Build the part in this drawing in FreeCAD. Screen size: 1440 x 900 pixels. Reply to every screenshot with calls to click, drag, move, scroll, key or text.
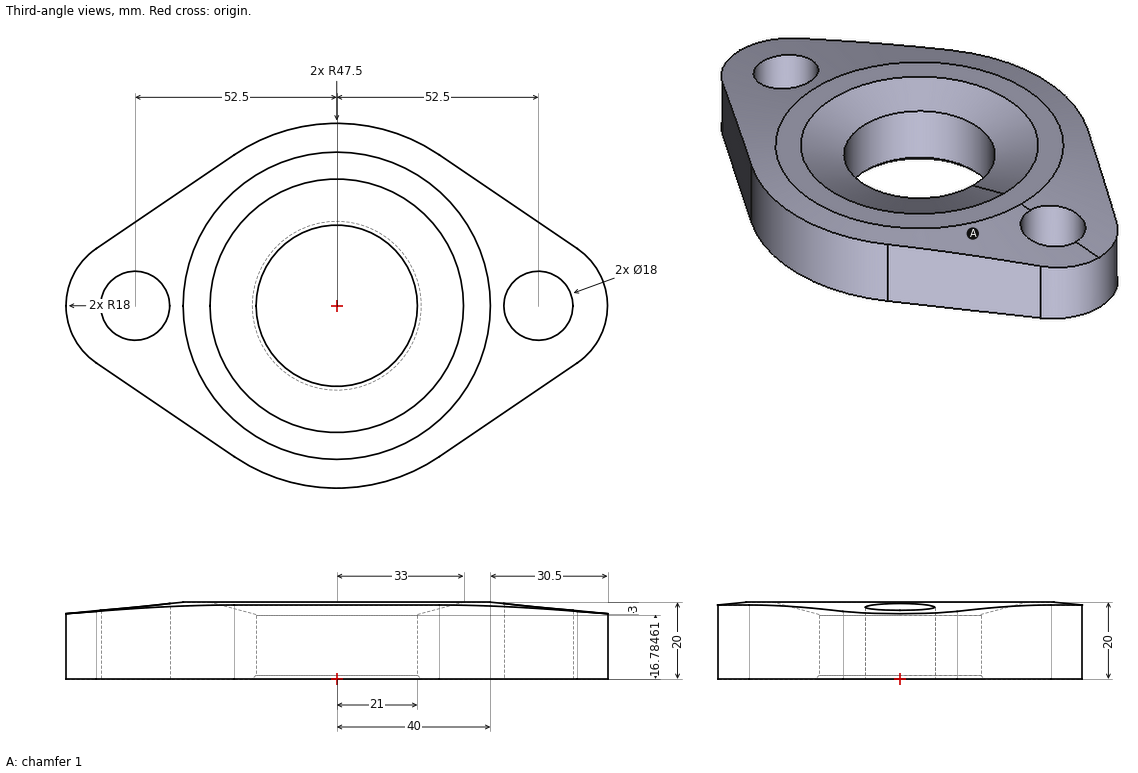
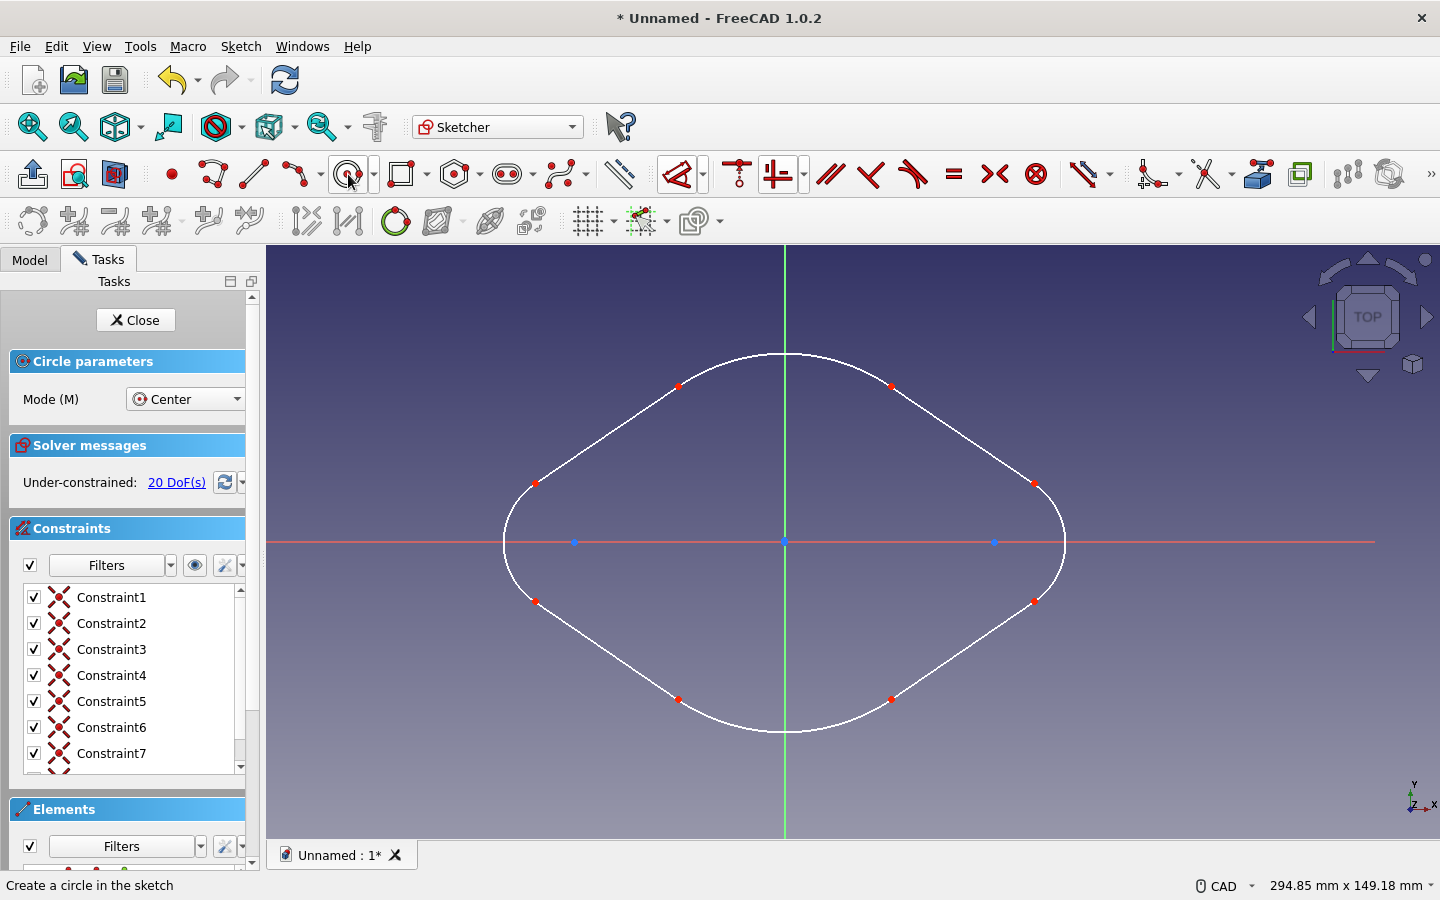
click(994, 542)
move(1019, 517)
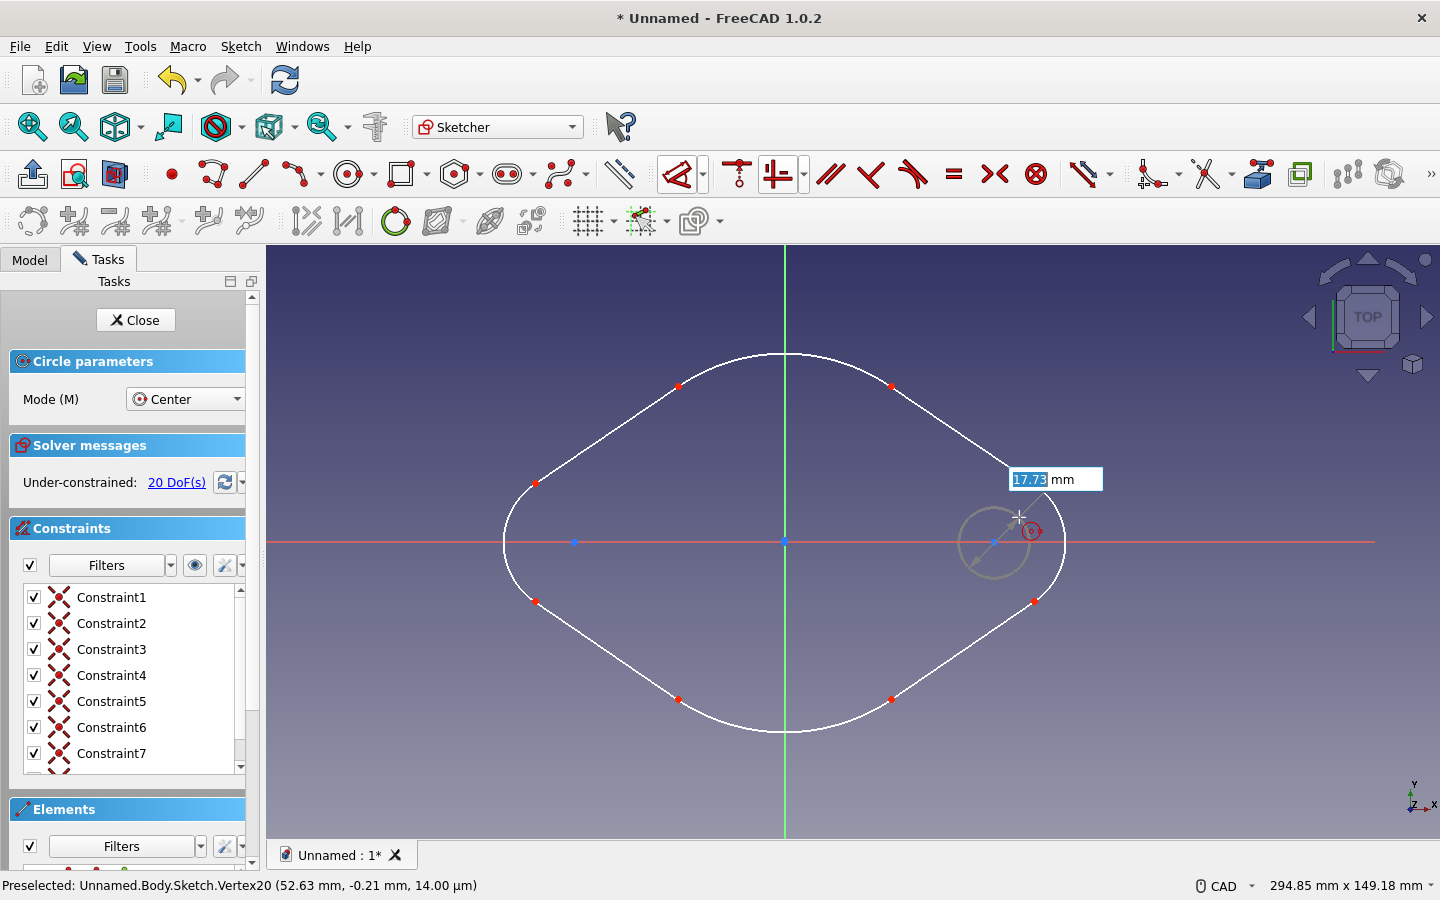
text(18)
key(Return)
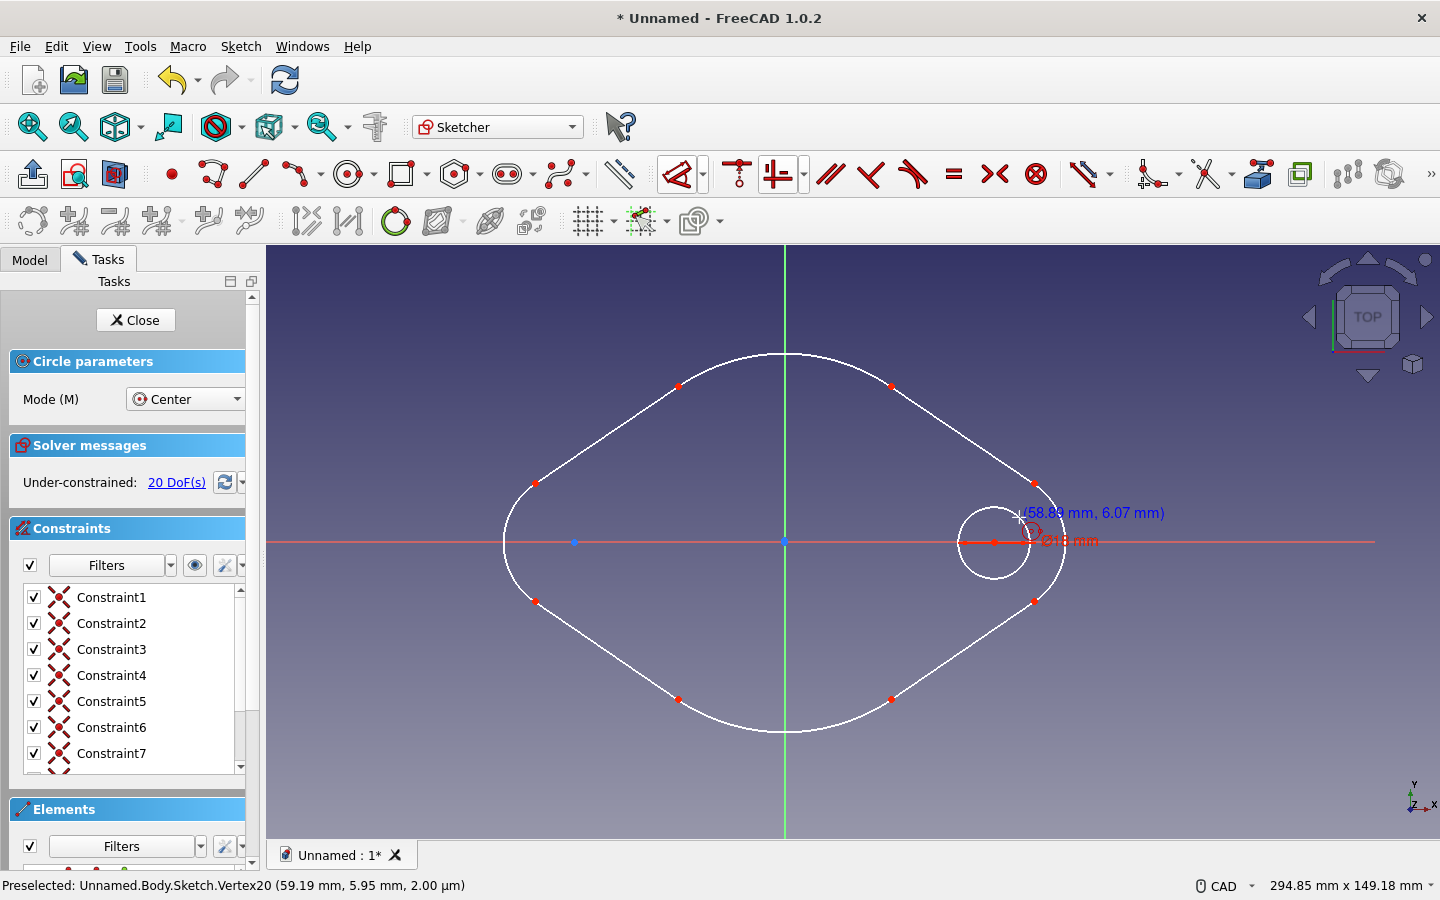
click(575, 542)
move(601, 517)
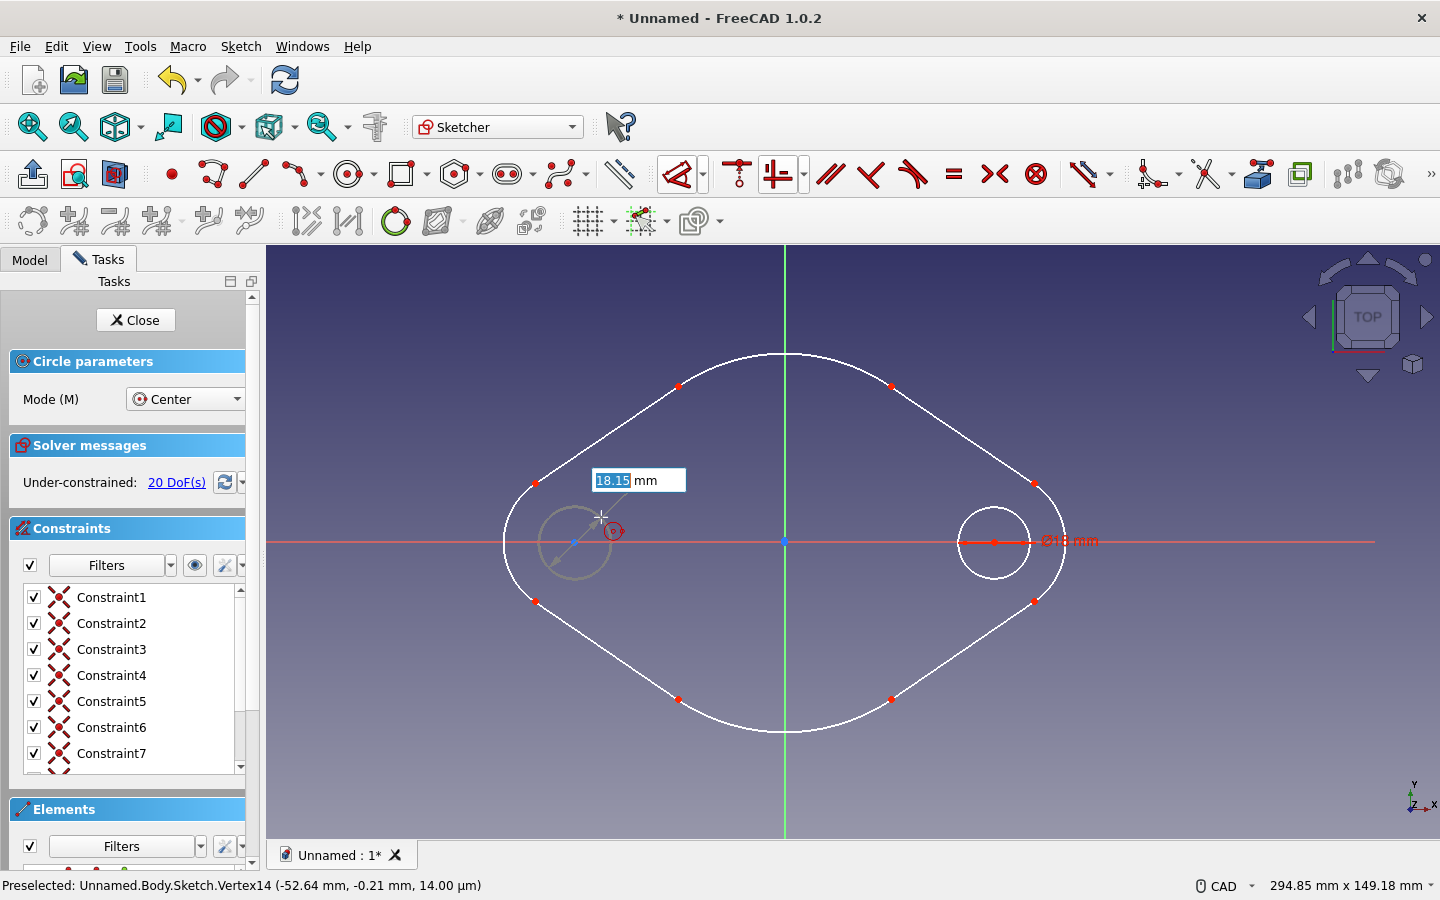
text(18)
key(Return)
key(Escape)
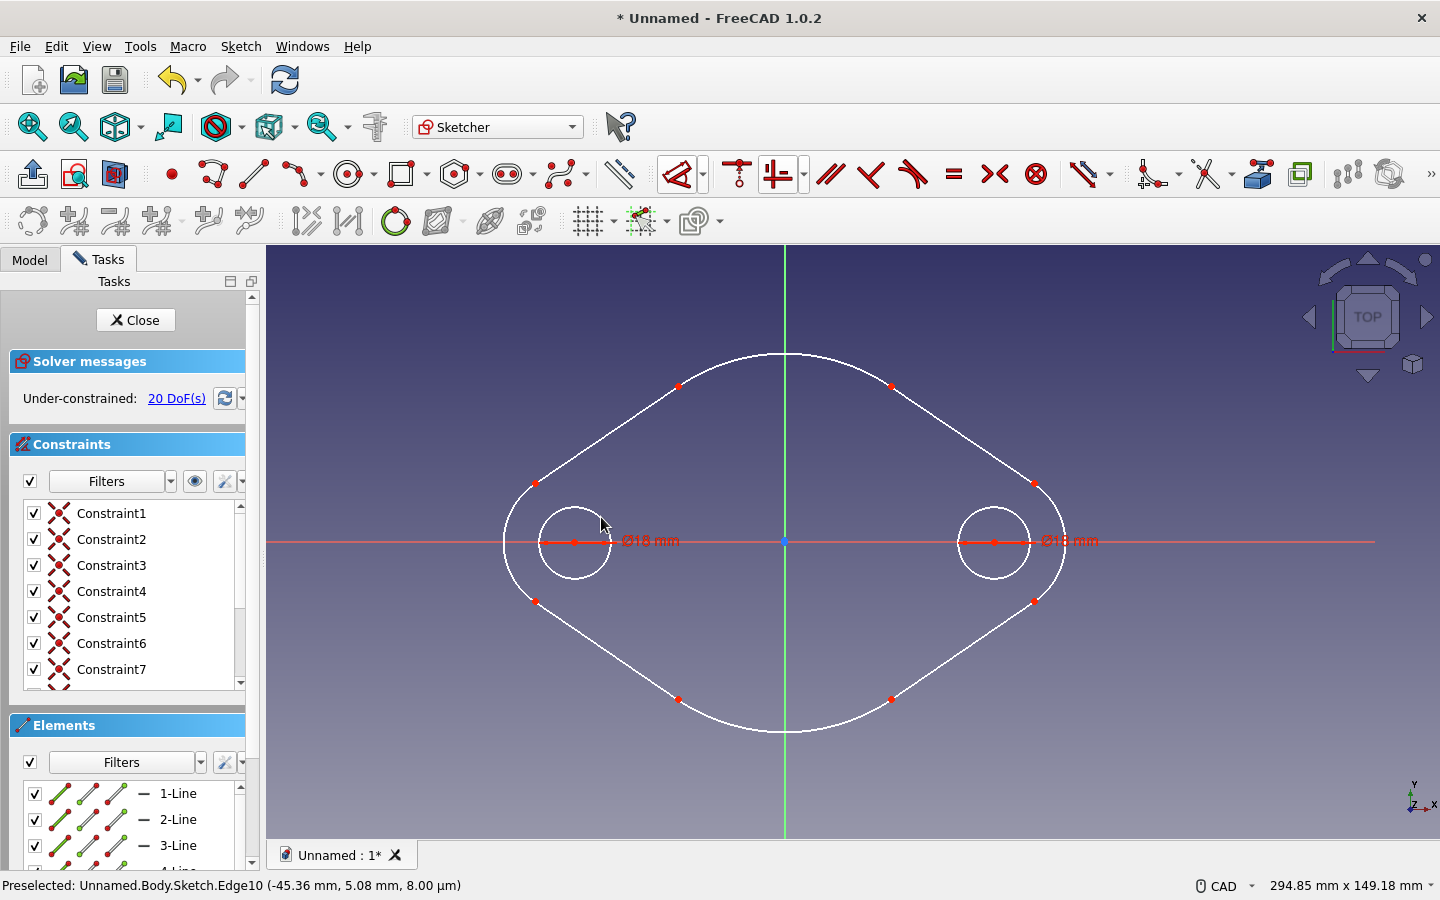
click(991, 455)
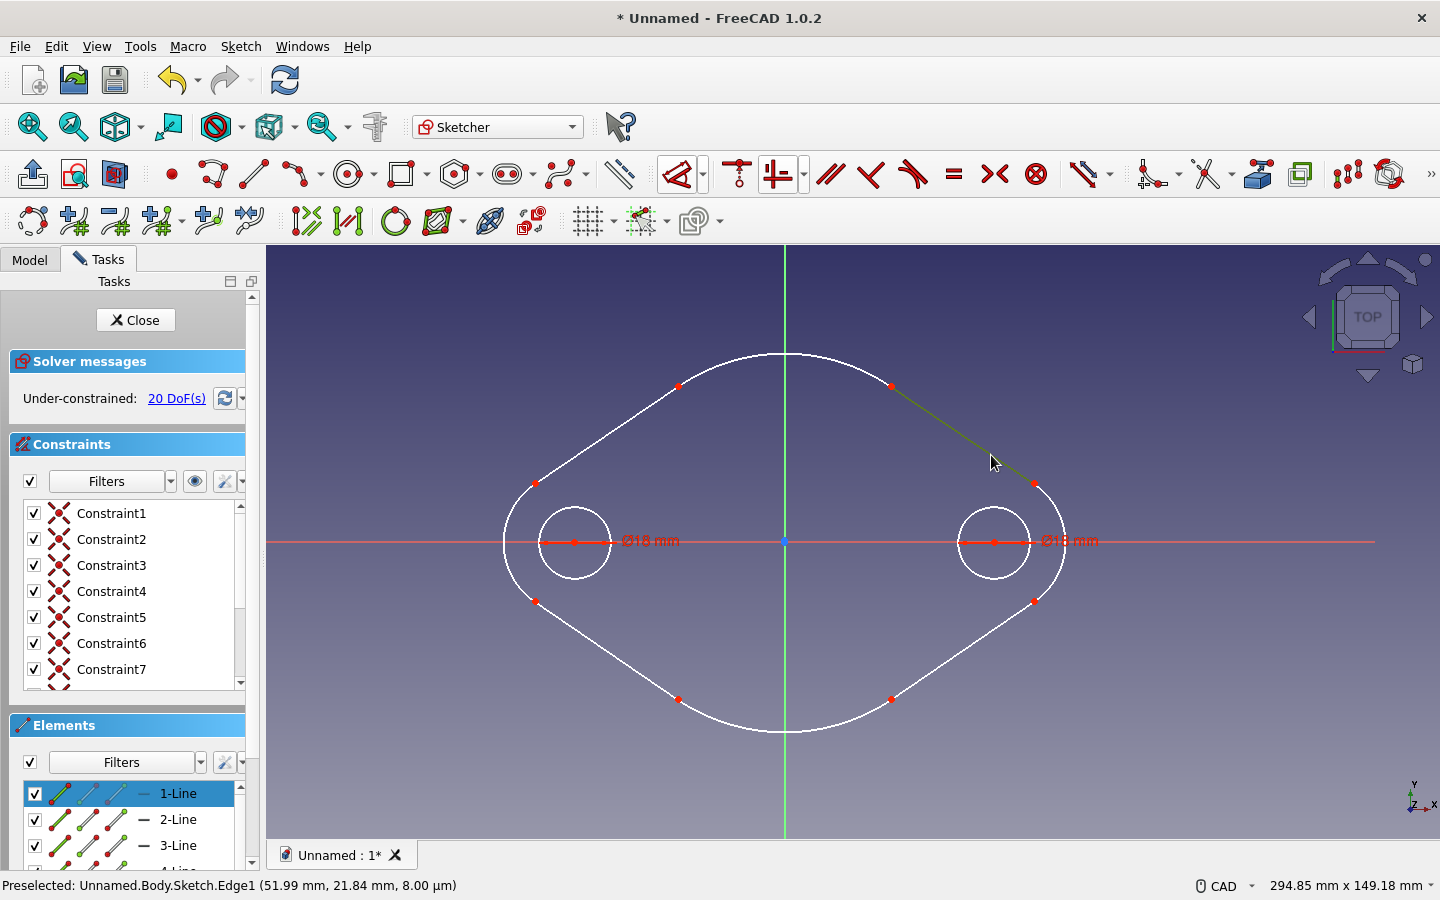
click(829, 359)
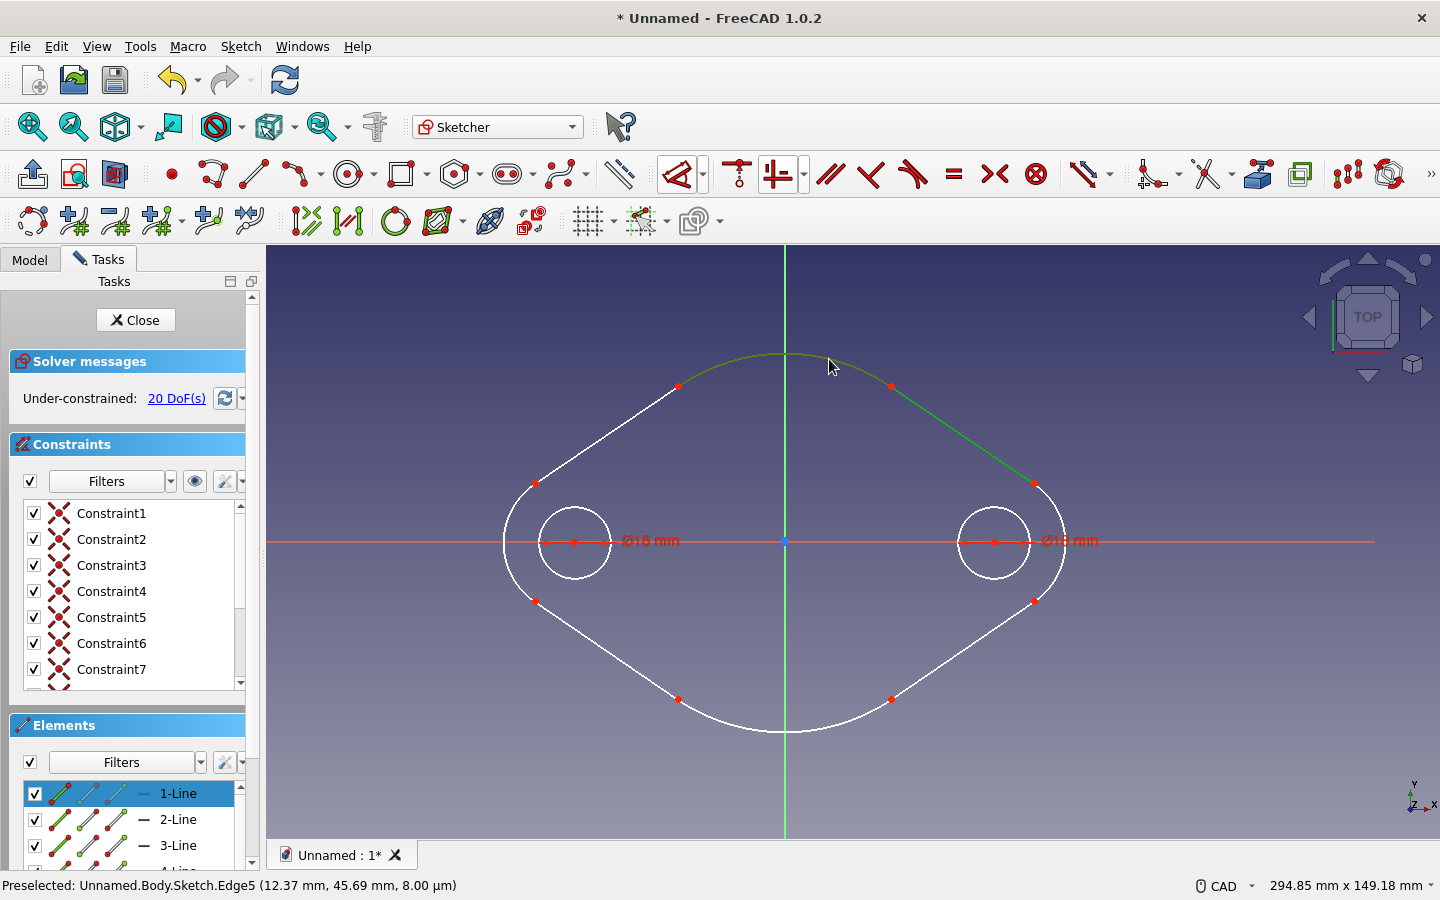
click(913, 174)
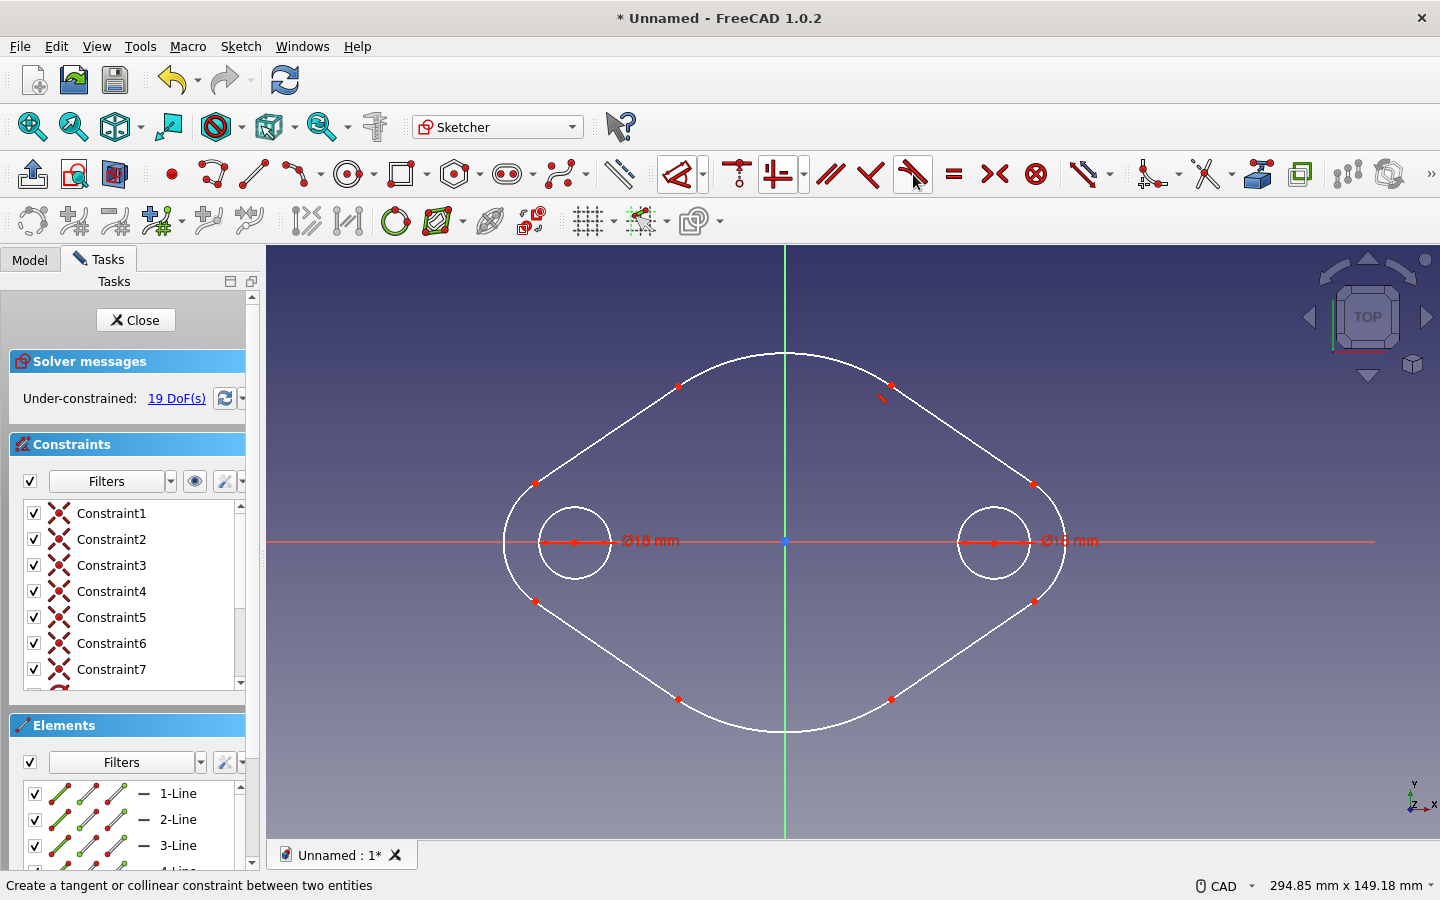
click(991, 455)